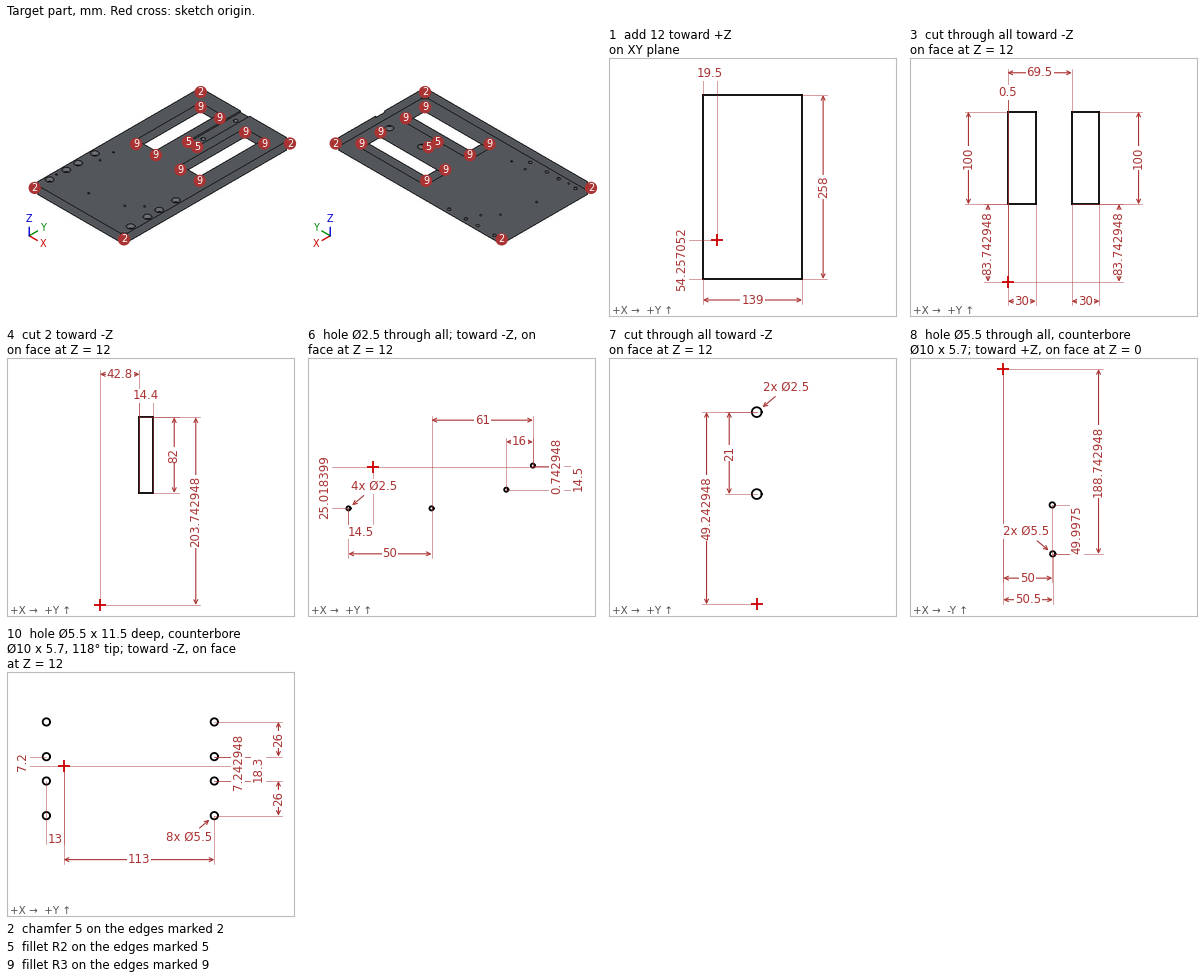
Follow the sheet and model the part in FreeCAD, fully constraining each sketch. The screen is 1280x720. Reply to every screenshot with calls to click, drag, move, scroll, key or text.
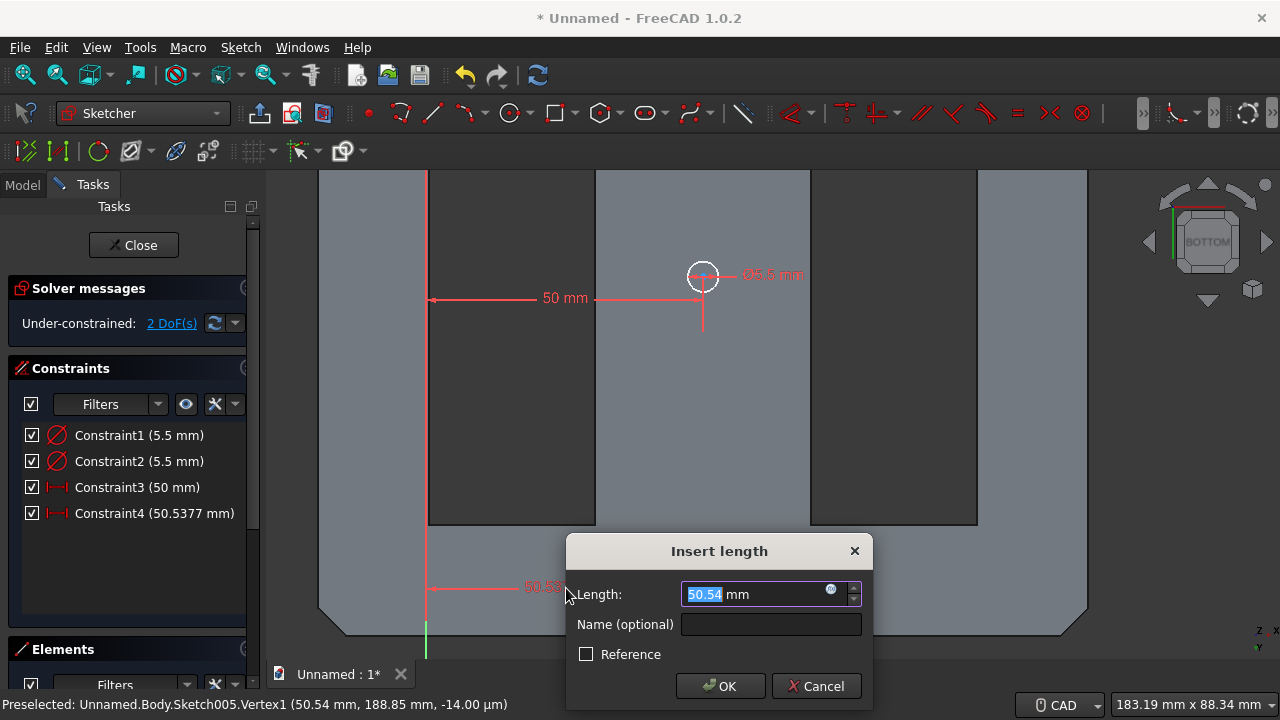
text(50.5)
key(Return)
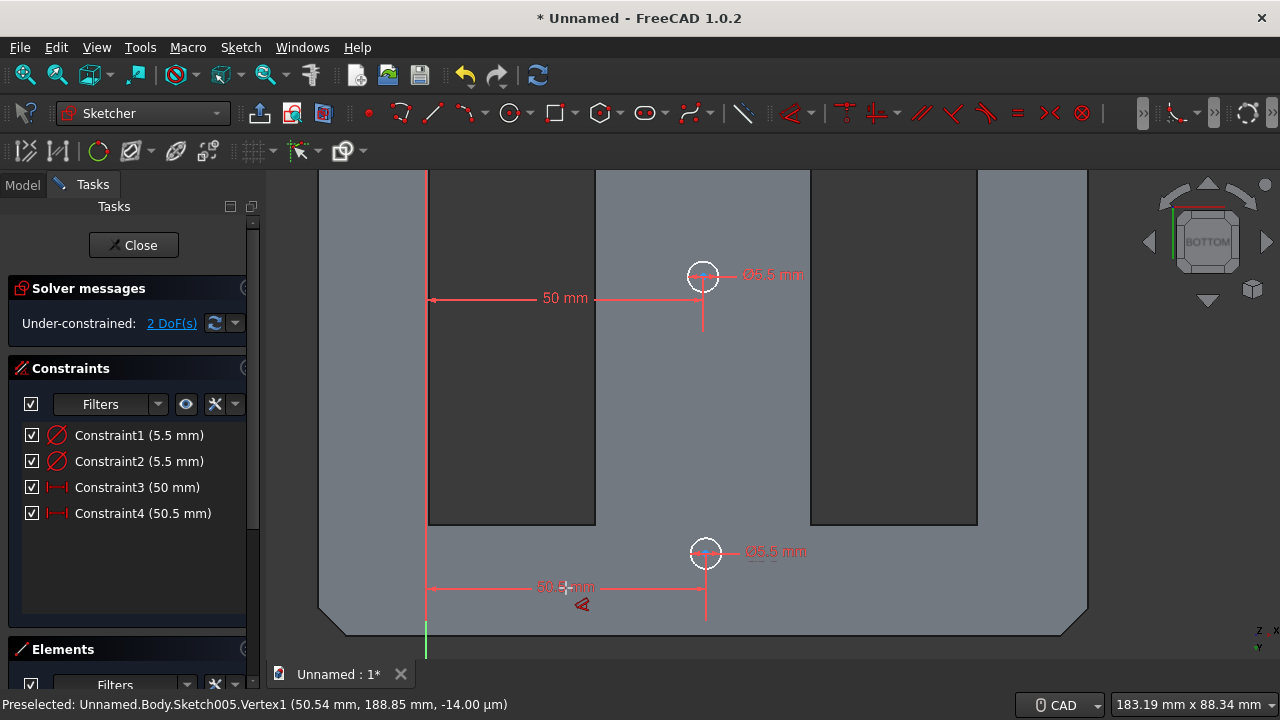
click(706, 554)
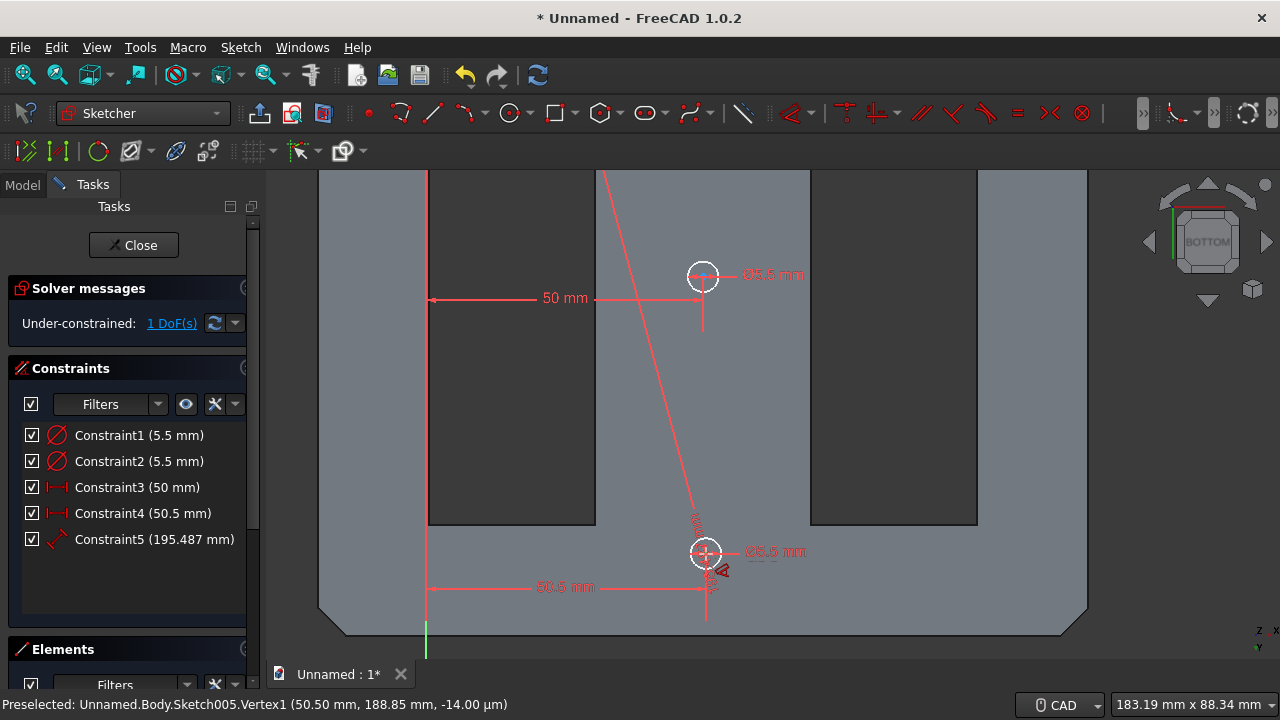
click(703, 277)
click(740, 415)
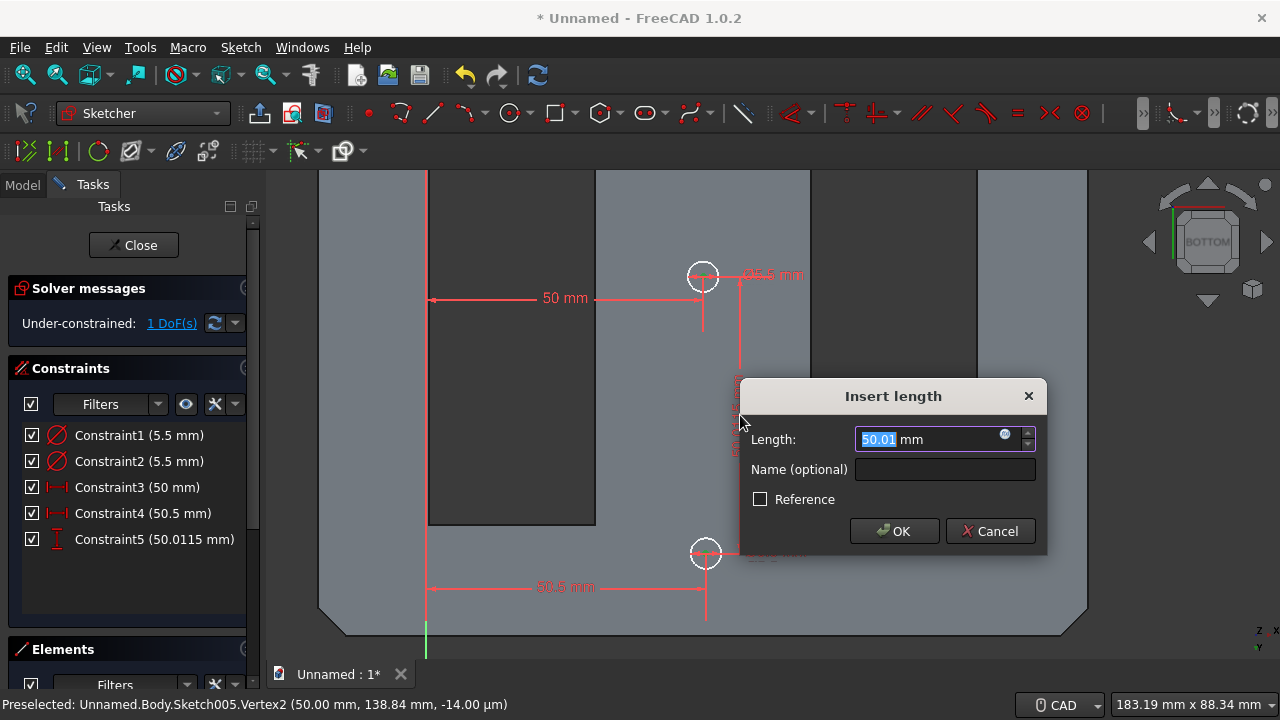
text(49.9975)
key(Return)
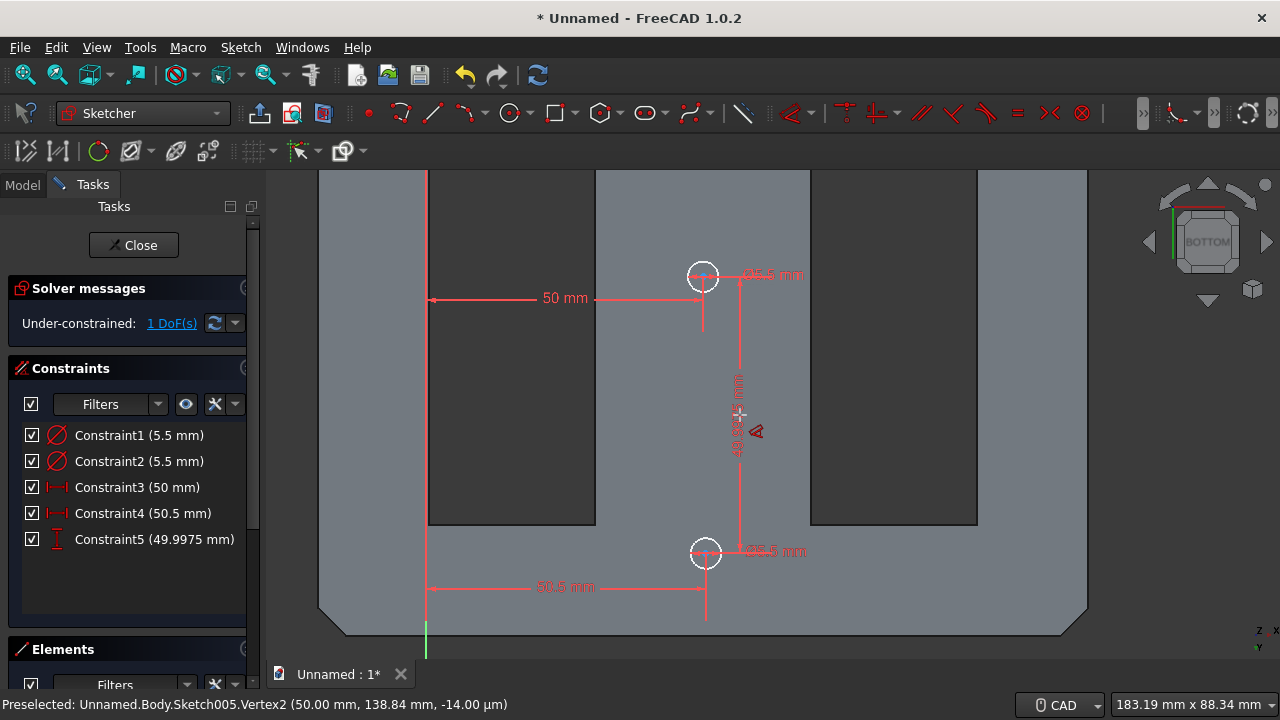
click(706, 553)
click(392, 376)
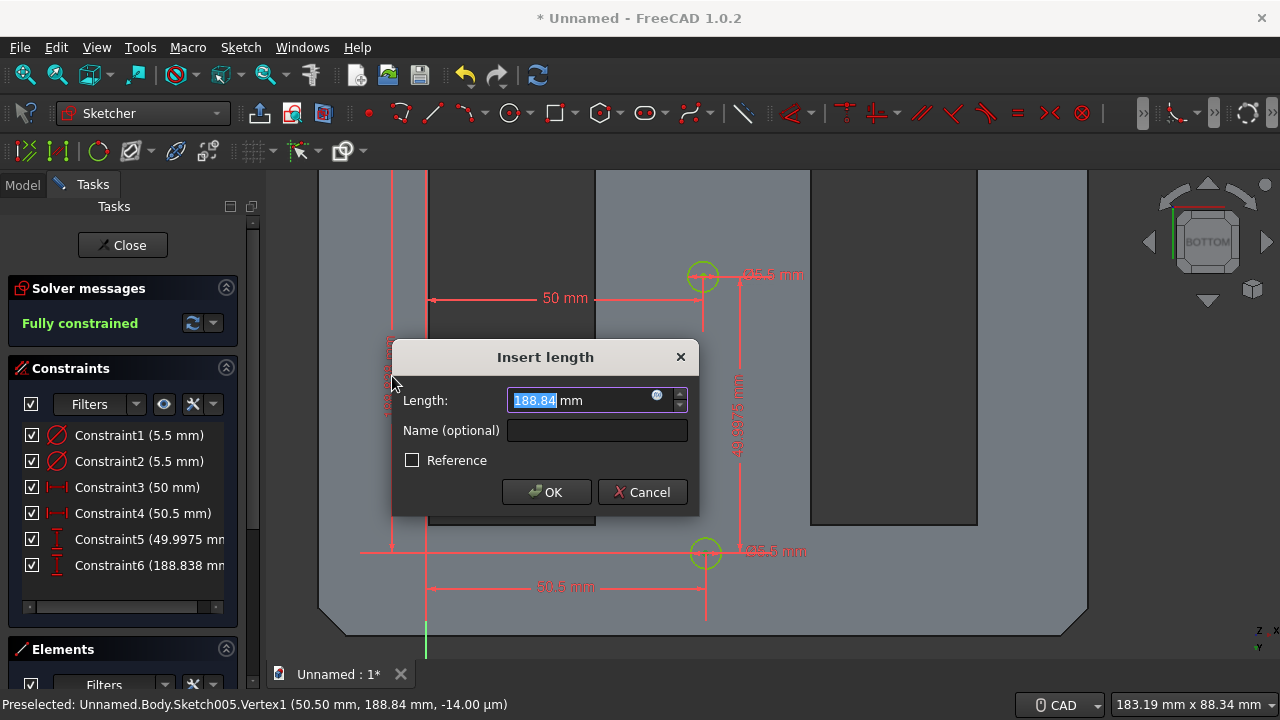
text(188.742948)
key(Return)
key(Escape)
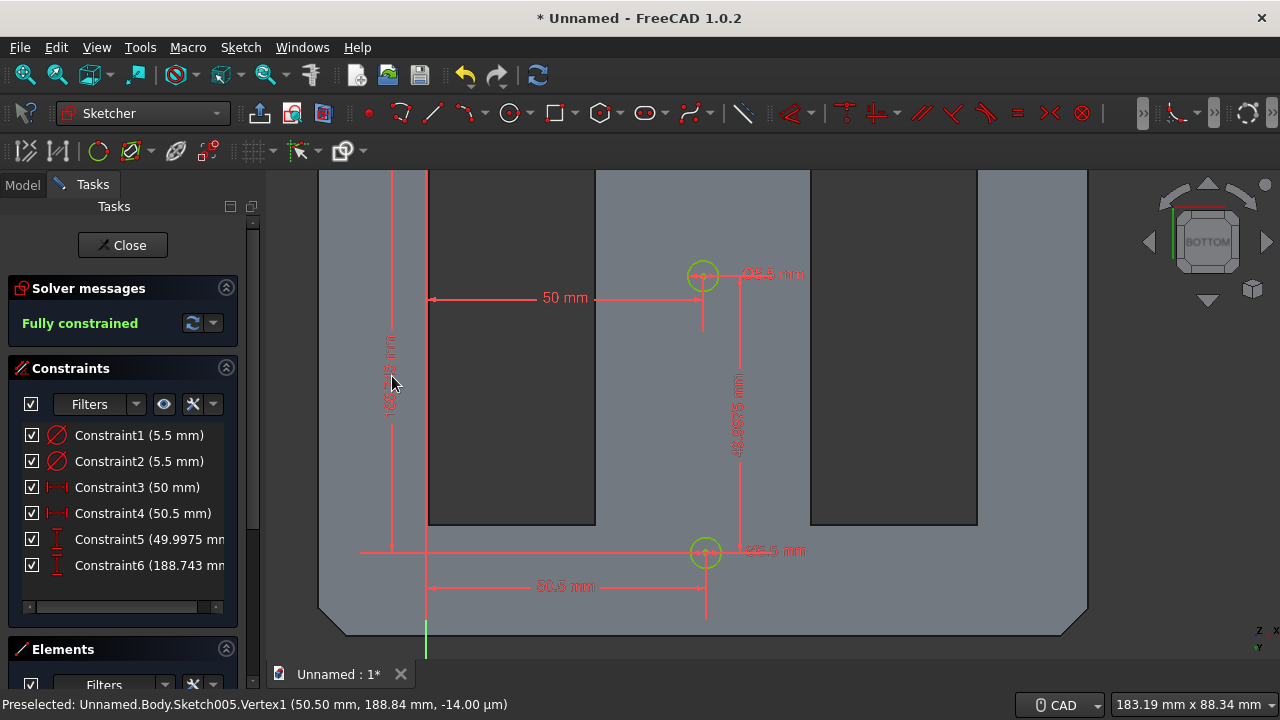
click(123, 245)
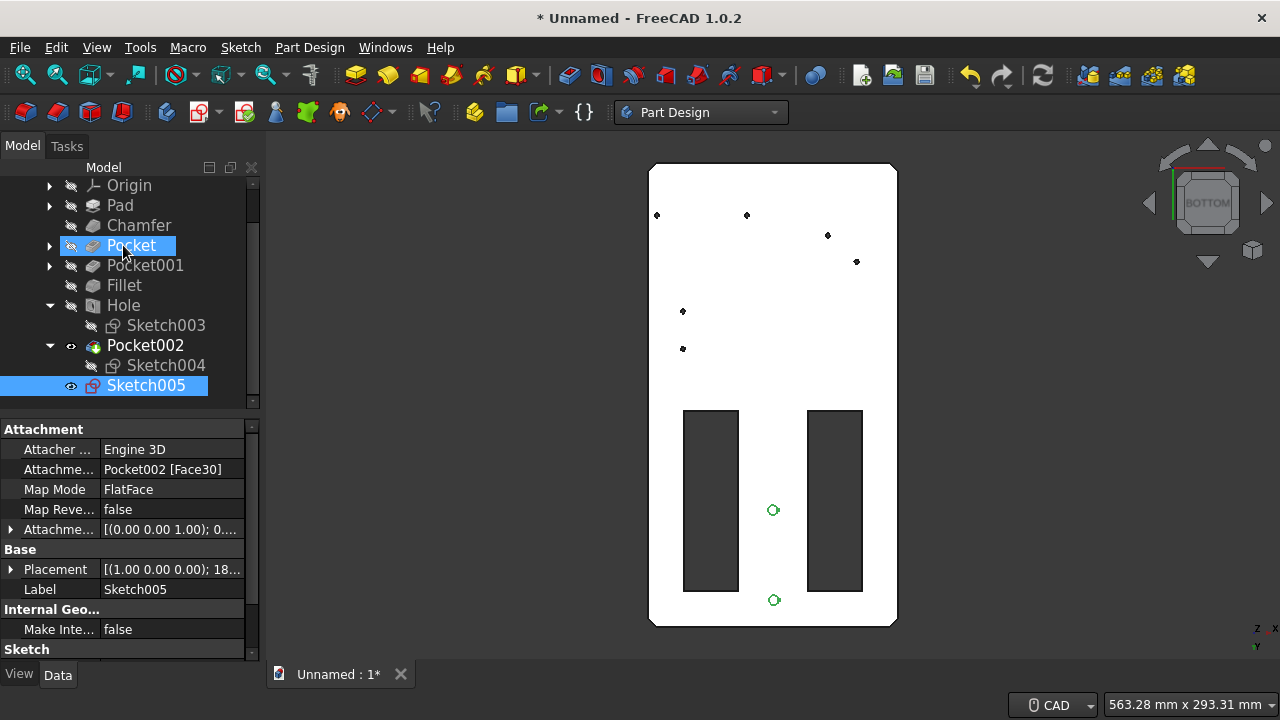
click(602, 76)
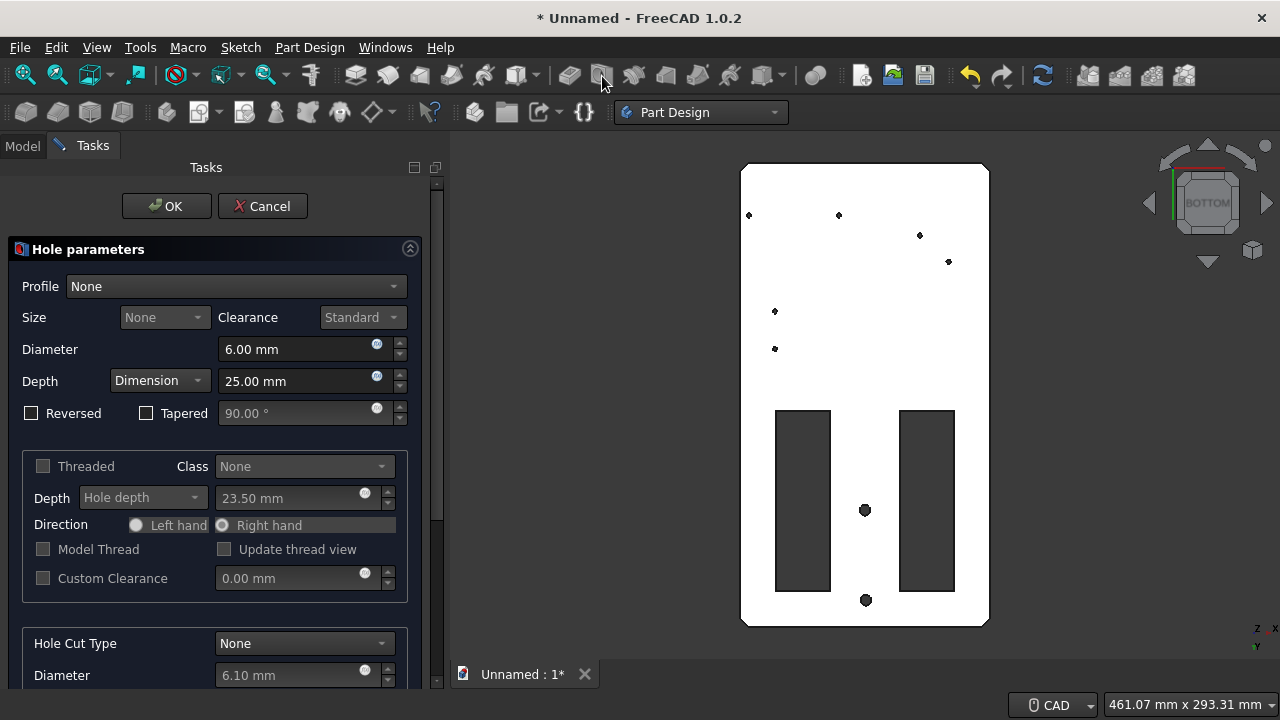
triple_click(305, 349)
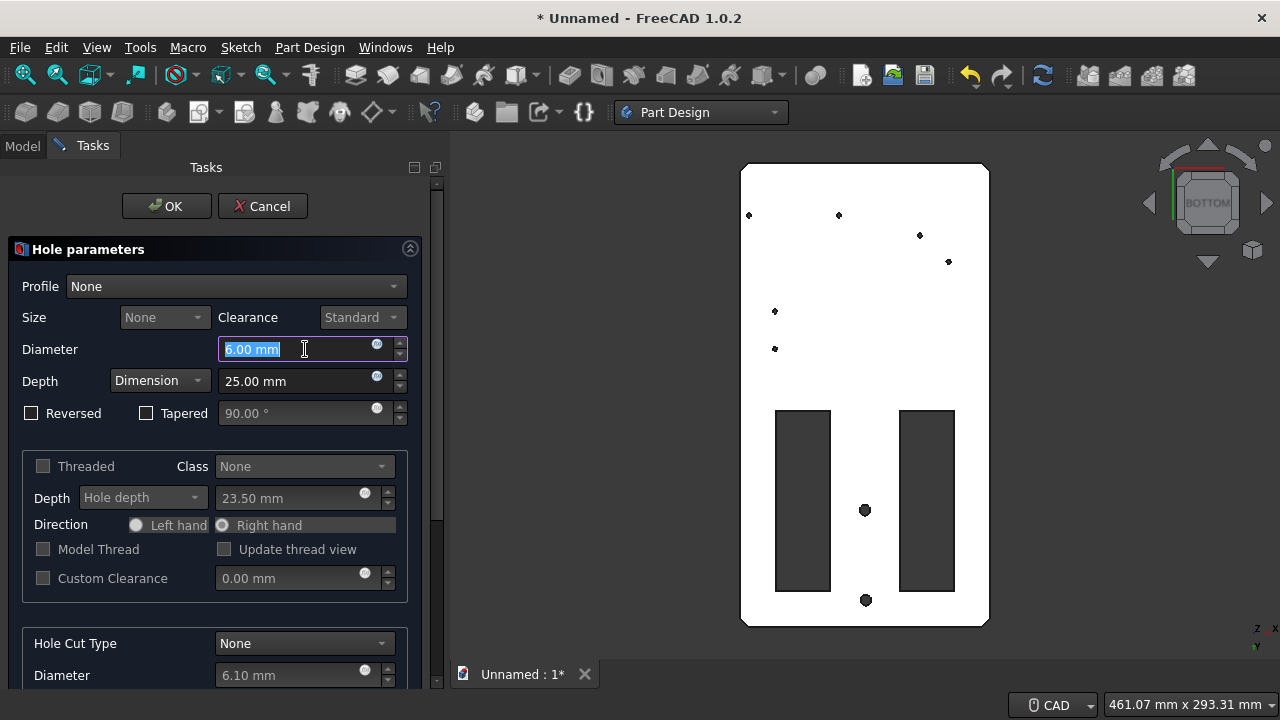
text(5.5)
key(Tab)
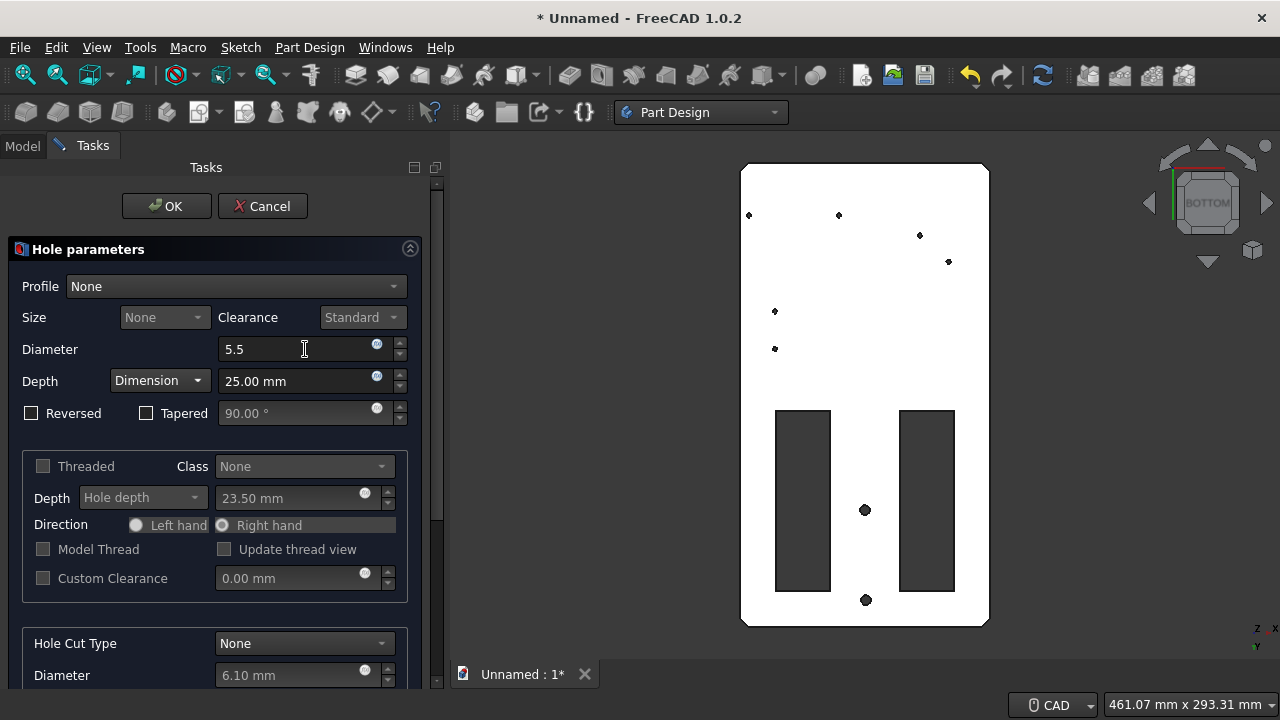
click(161, 380)